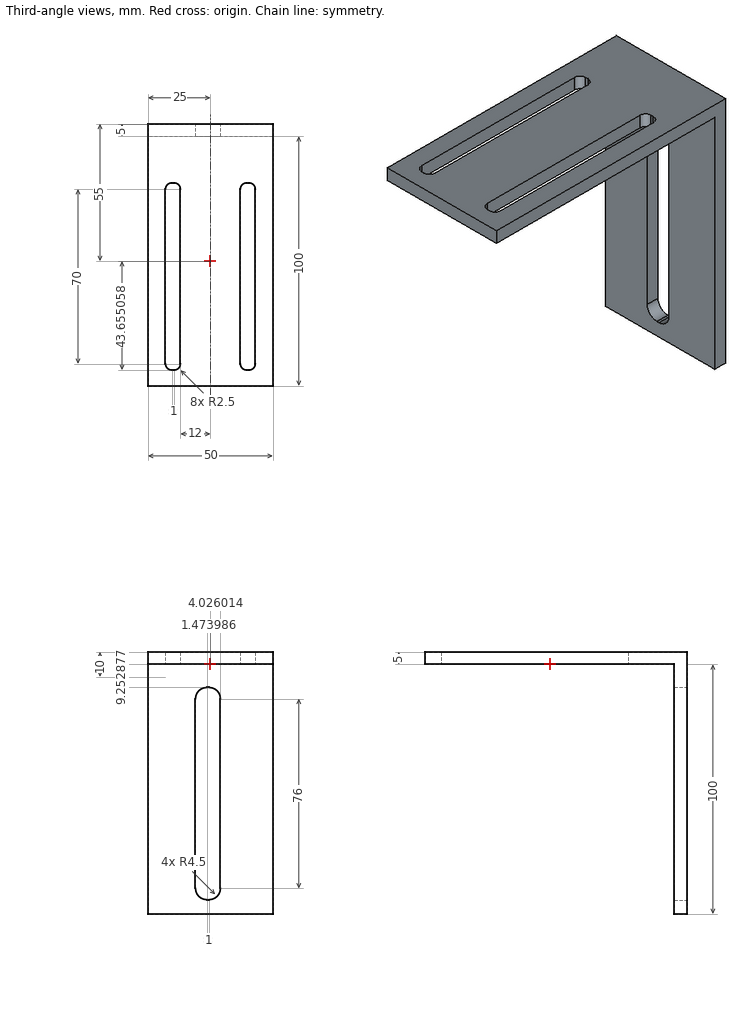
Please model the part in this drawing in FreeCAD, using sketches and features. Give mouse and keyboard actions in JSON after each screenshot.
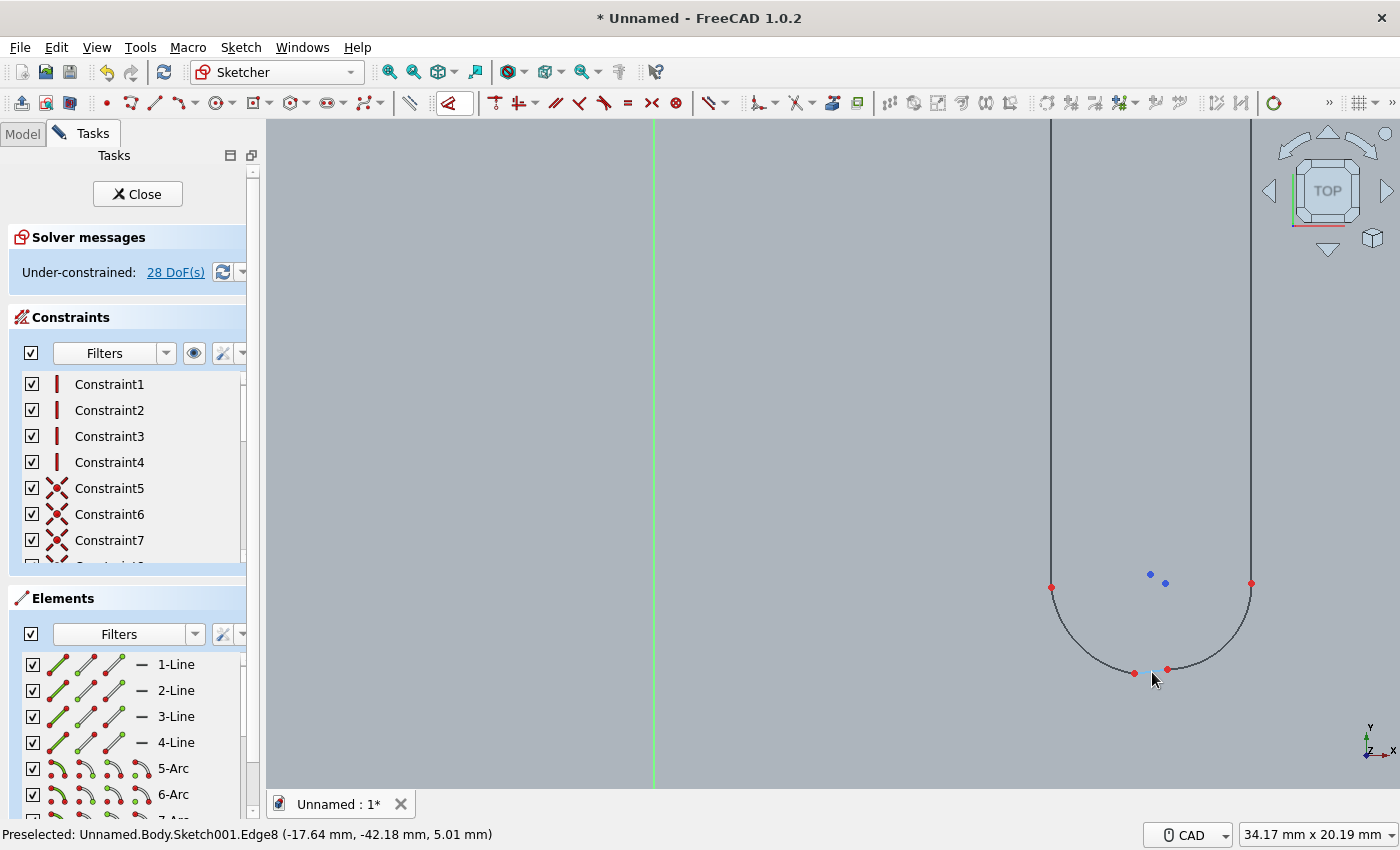
{"action": "left_click", "coordinate": [1151, 672]}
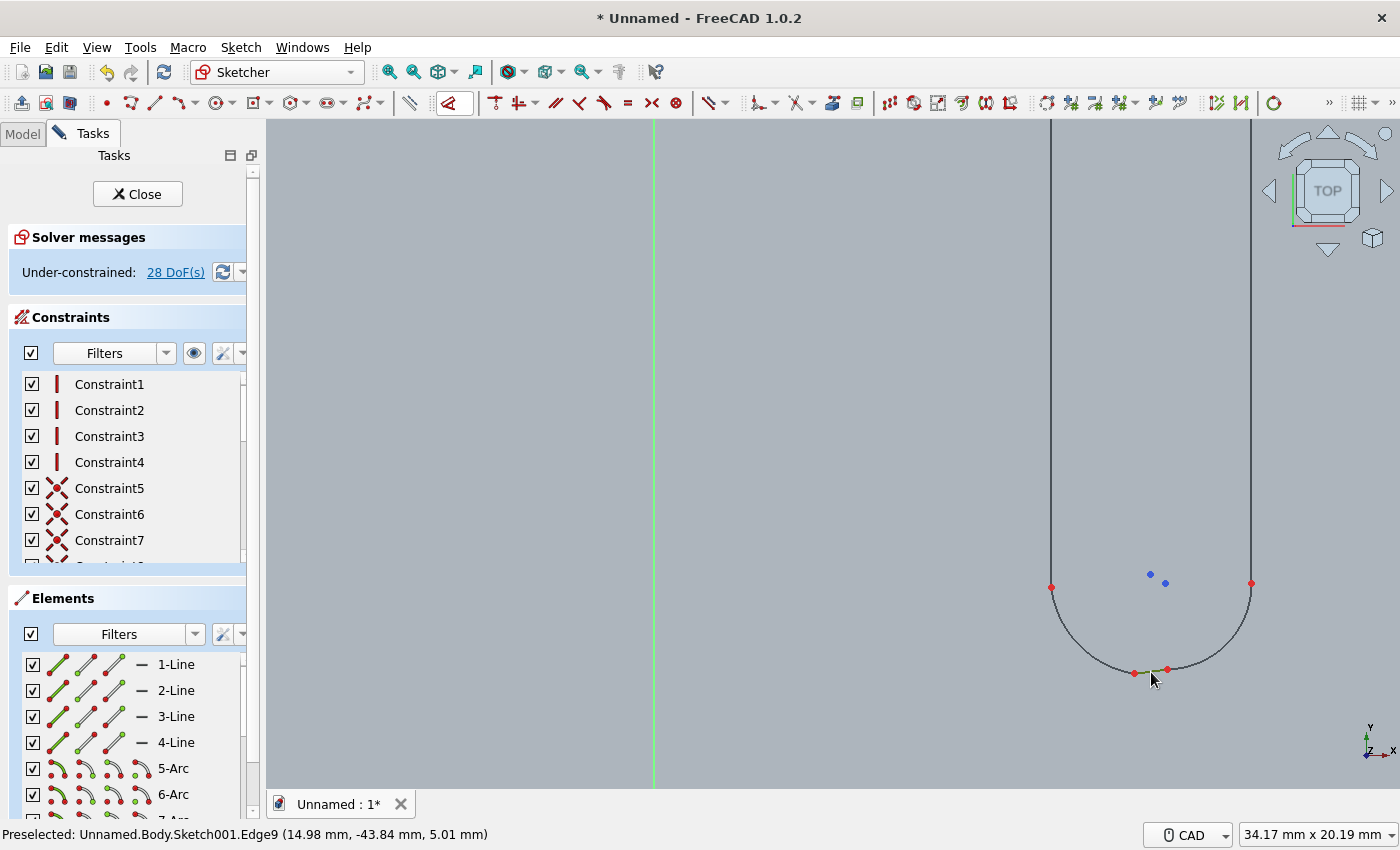
{"action": "left_click", "coordinate": [1206, 660]}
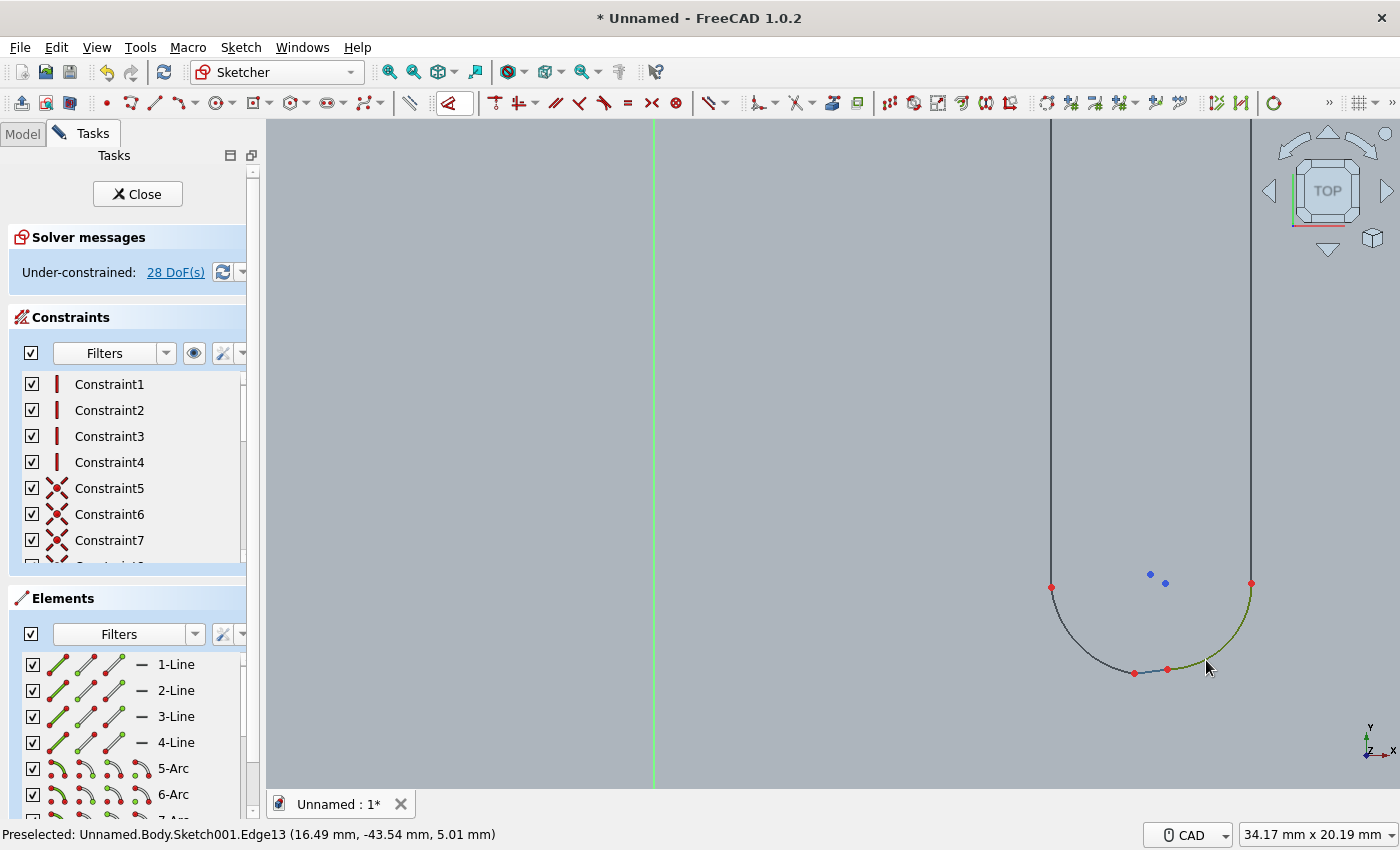
{"action": "key", "text": "t"}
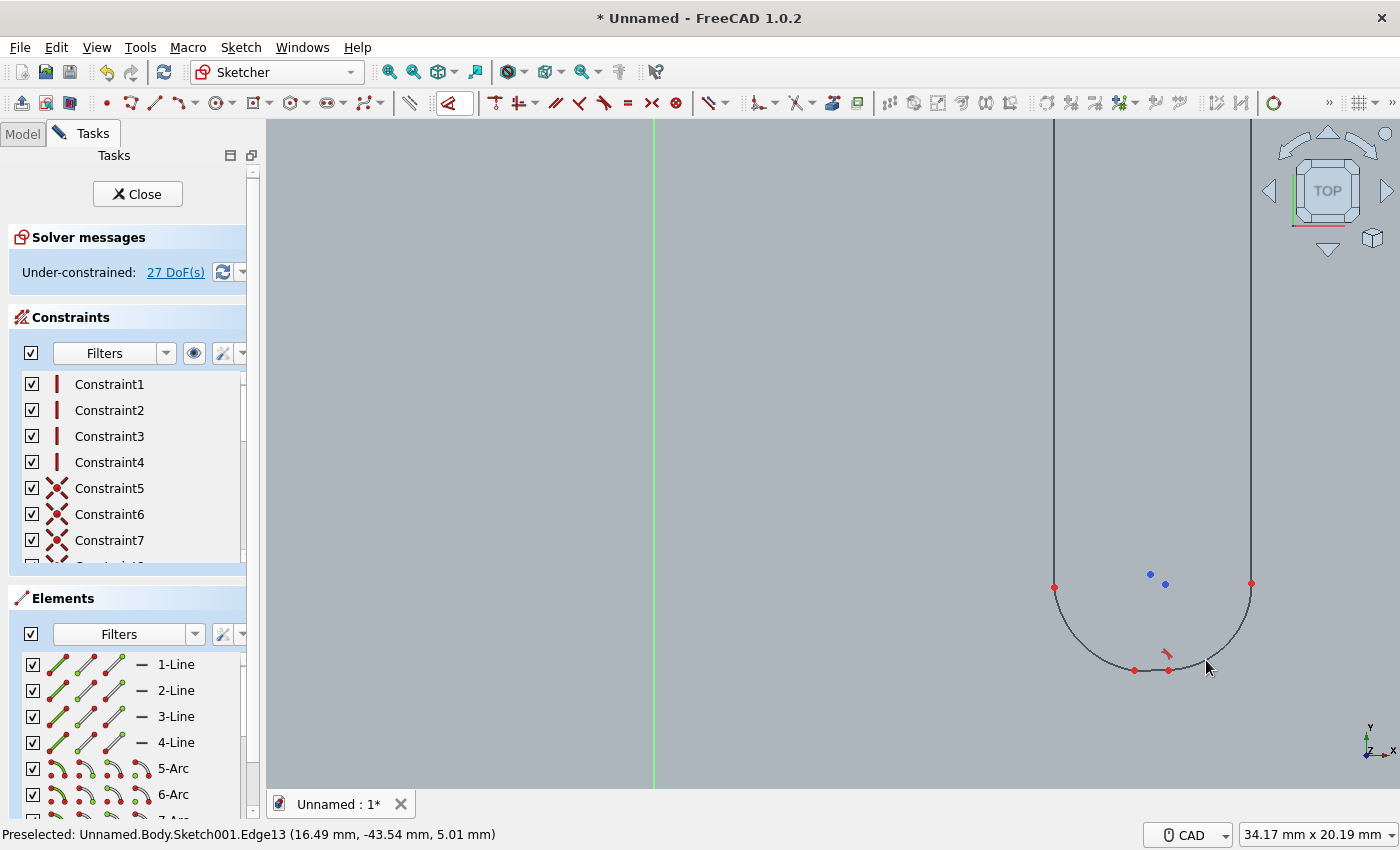
{"action": "scroll", "coordinate": [1145, 671], "scroll_direction": "up", "scroll_amount": 2}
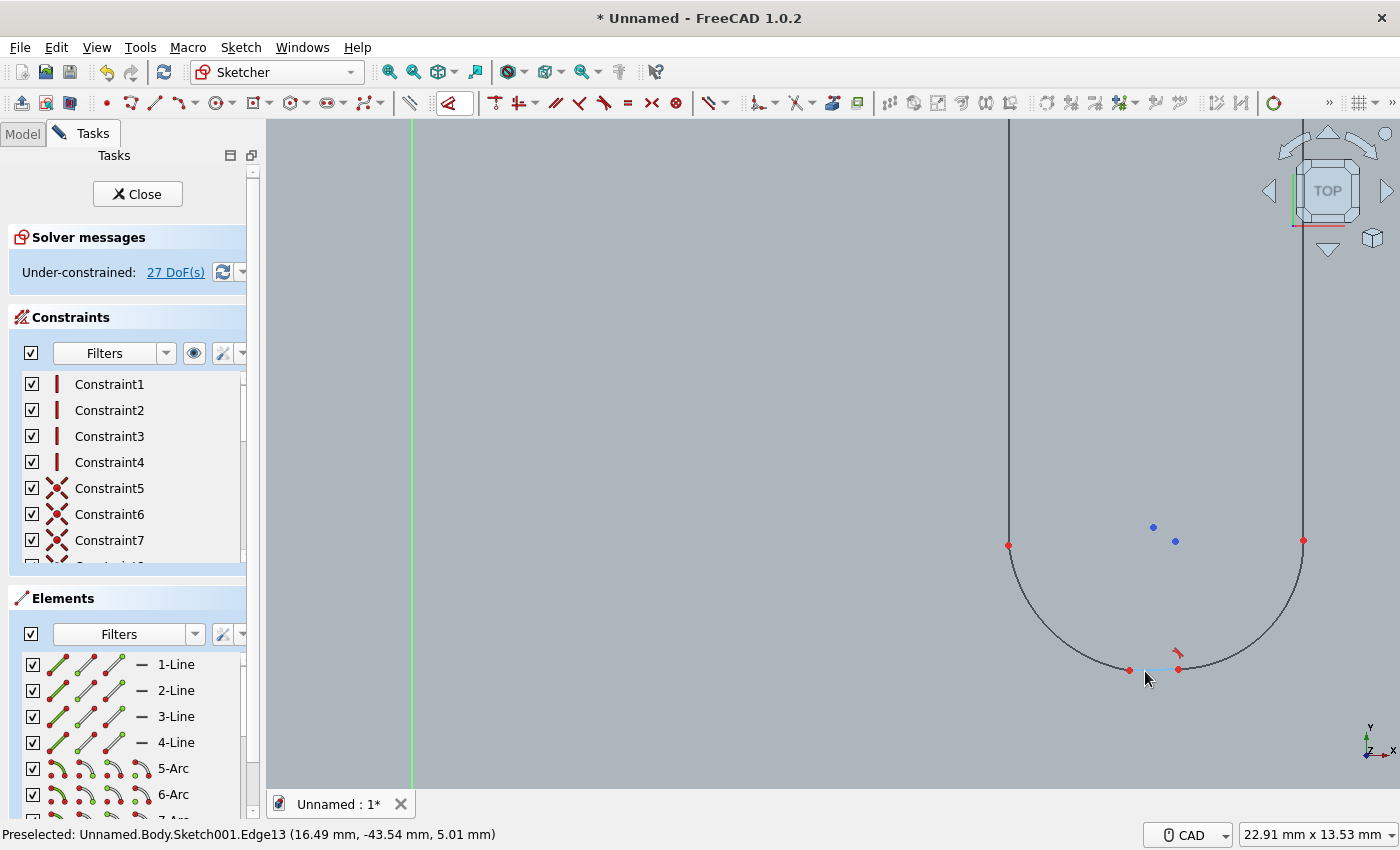
{"action": "left_click", "coordinate": [1144, 670]}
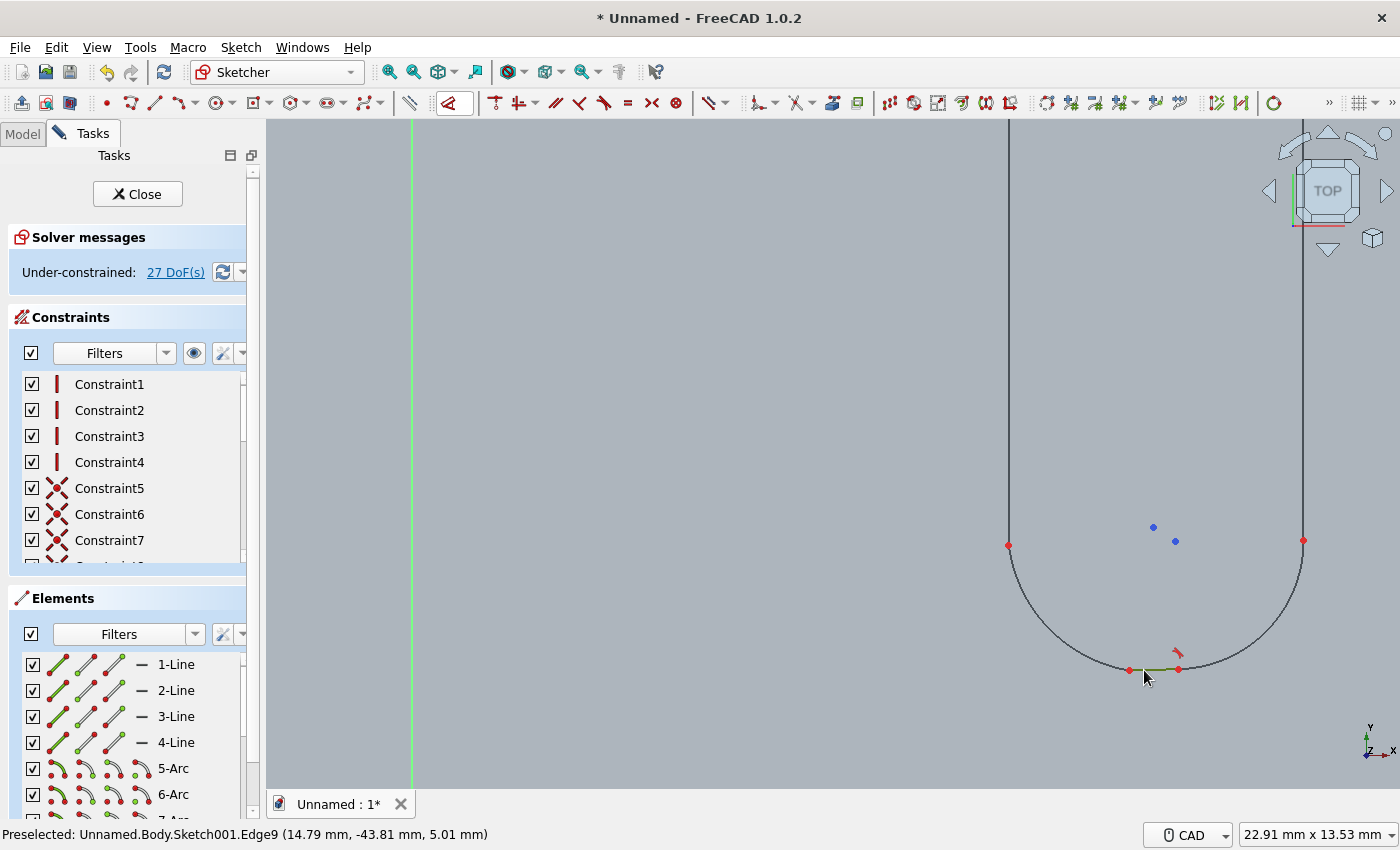
{"action": "scroll", "coordinate": [808, 659], "scroll_direction": "down", "scroll_amount": 11}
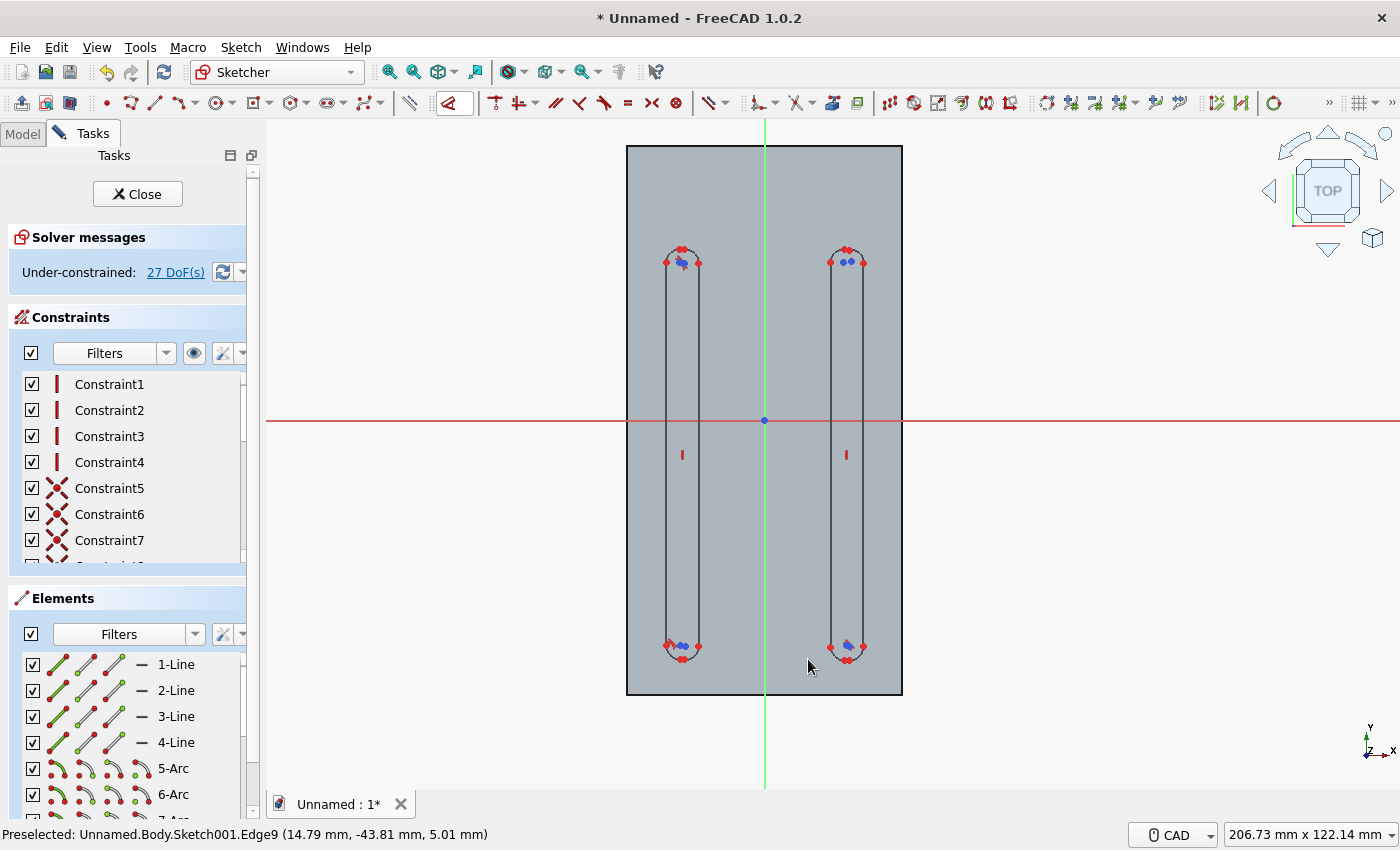
{"action": "scroll", "coordinate": [833, 653], "scroll_direction": "up", "scroll_amount": 5}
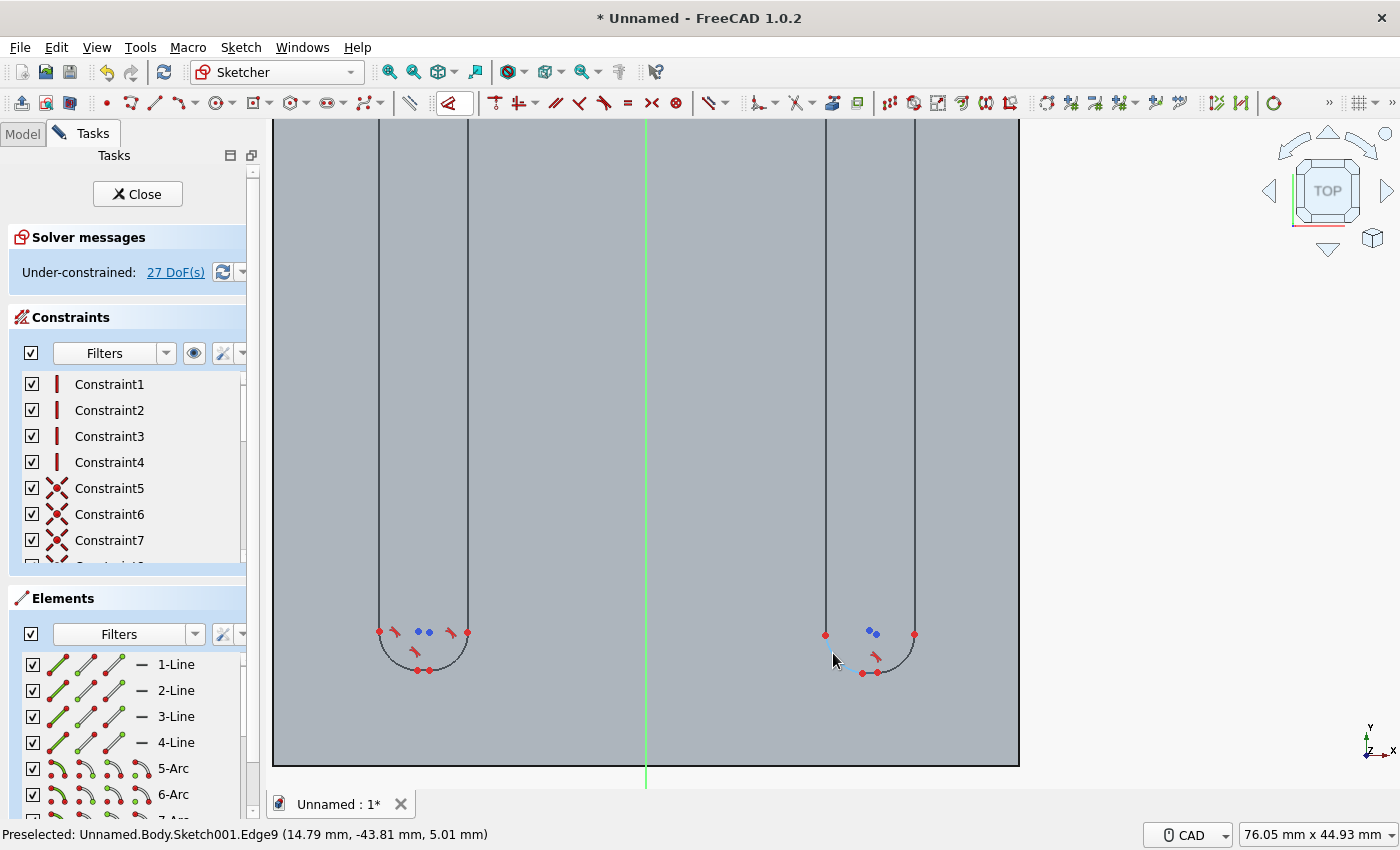
{"action": "left_click", "coordinate": [831, 652]}